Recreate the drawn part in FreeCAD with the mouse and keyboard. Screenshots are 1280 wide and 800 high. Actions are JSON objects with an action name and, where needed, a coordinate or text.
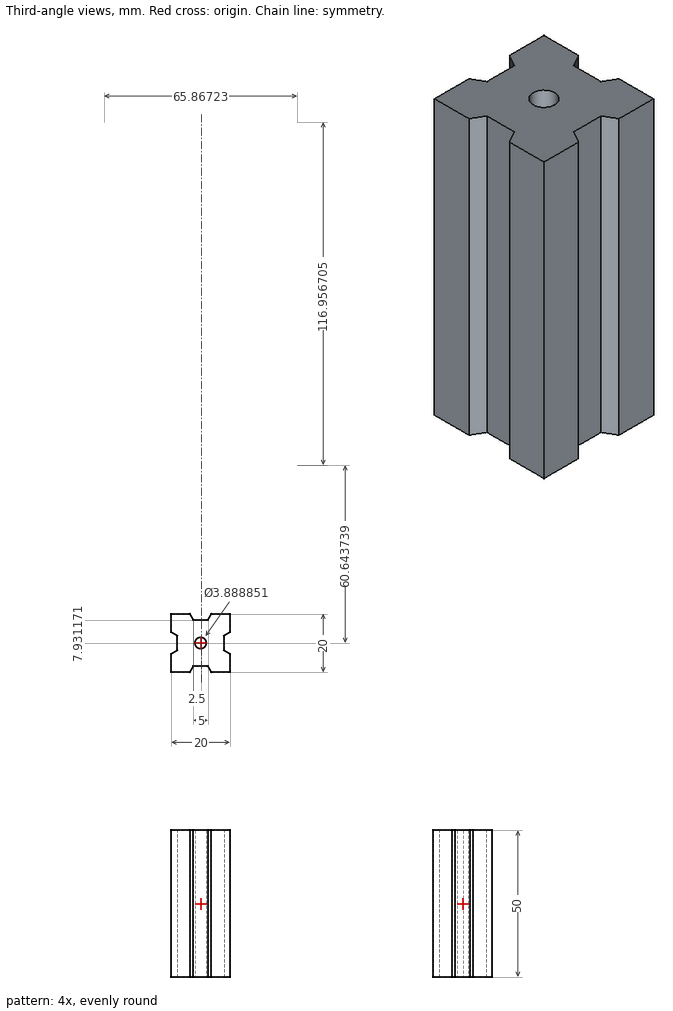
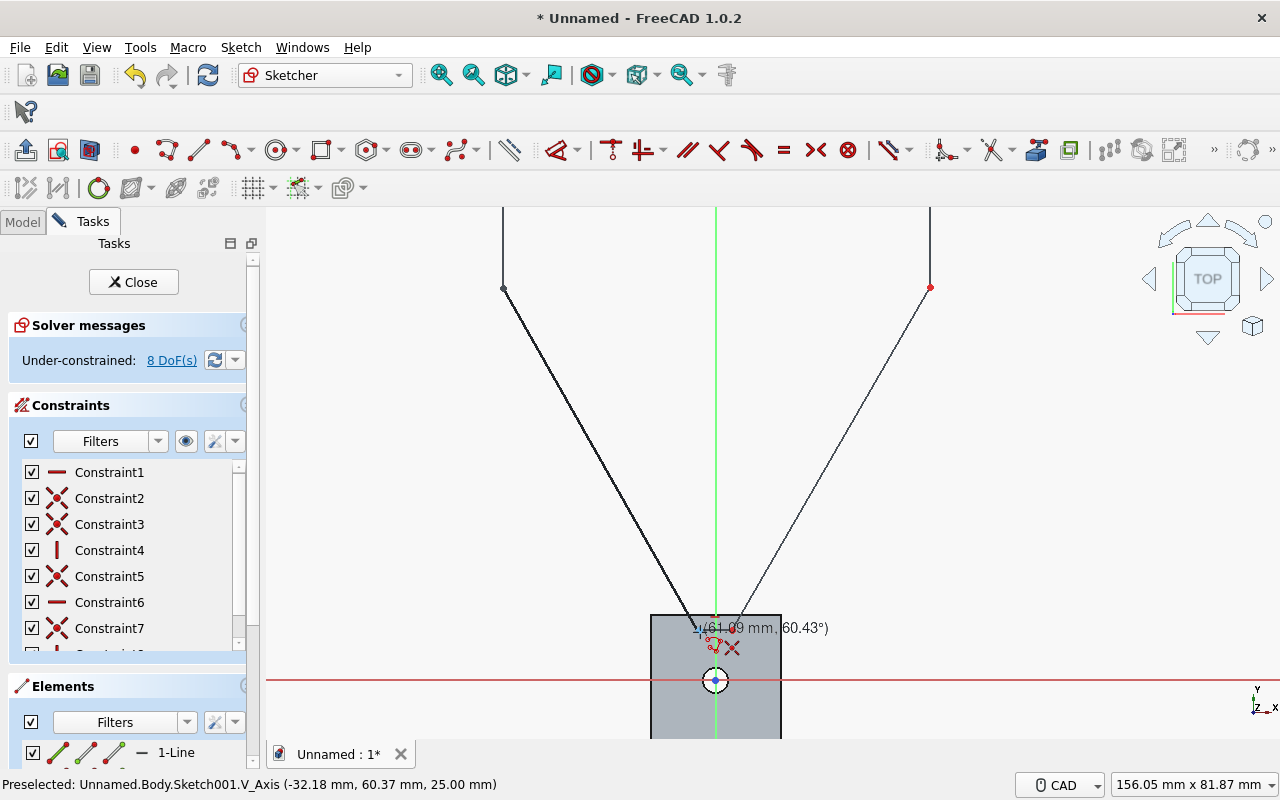
{"action": "left_click", "coordinate": [699, 630]}
{"action": "key", "text": "Escape"}
{"action": "key", "text": "Escape"}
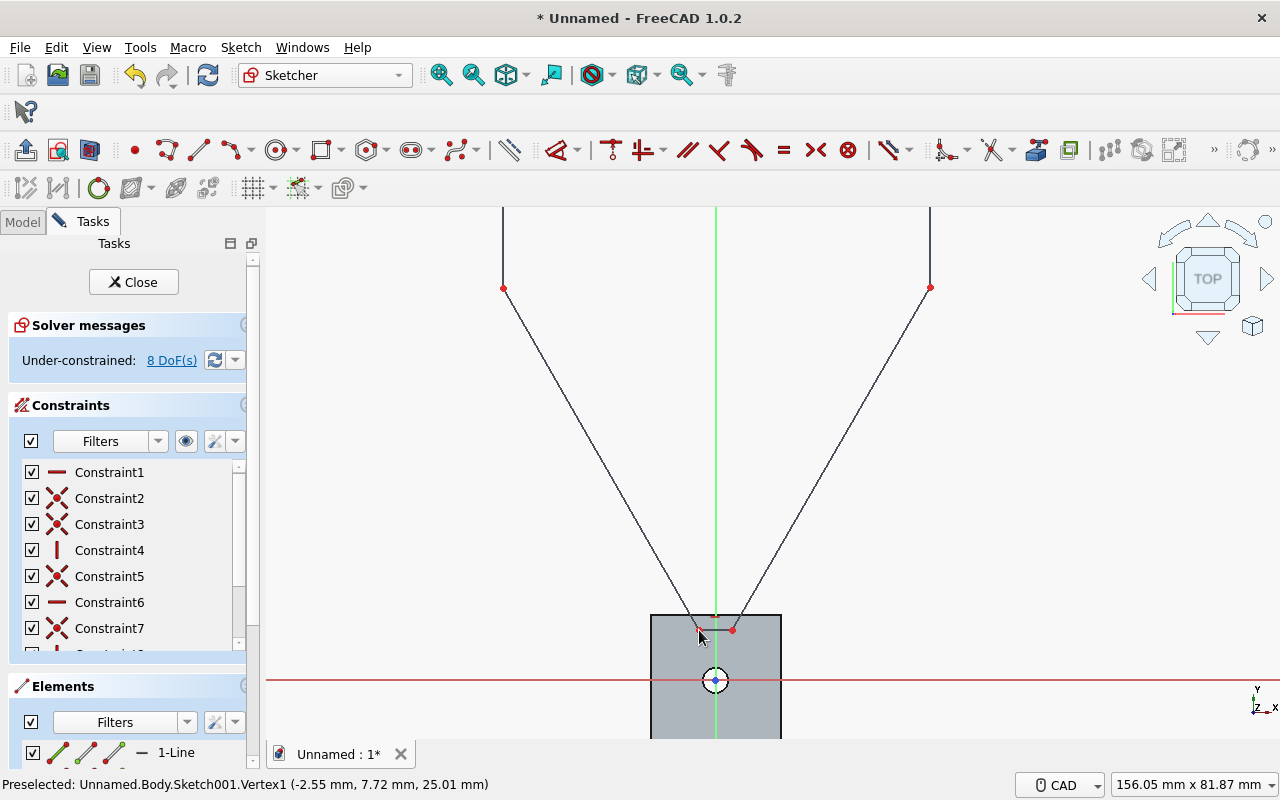
{"action": "left_click", "coordinate": [930, 287]}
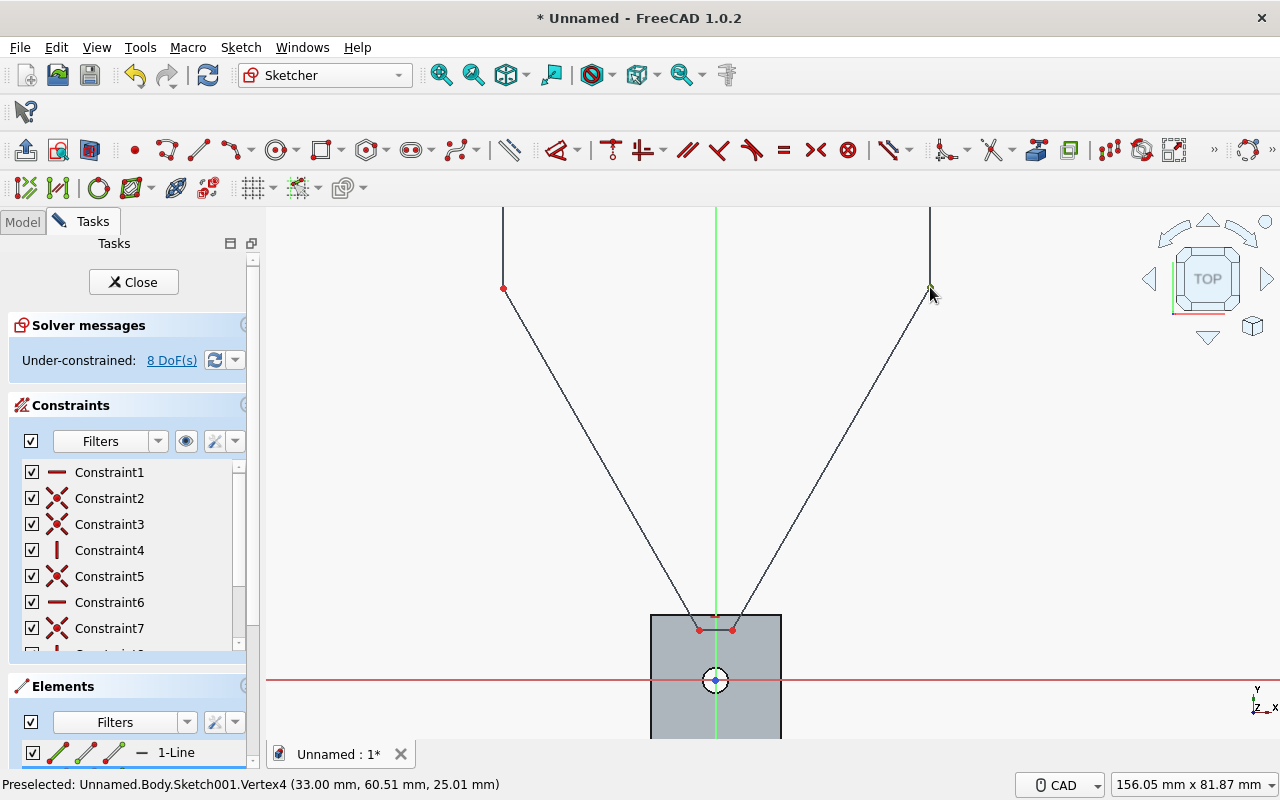
{"action": "left_click", "coordinate": [503, 288]}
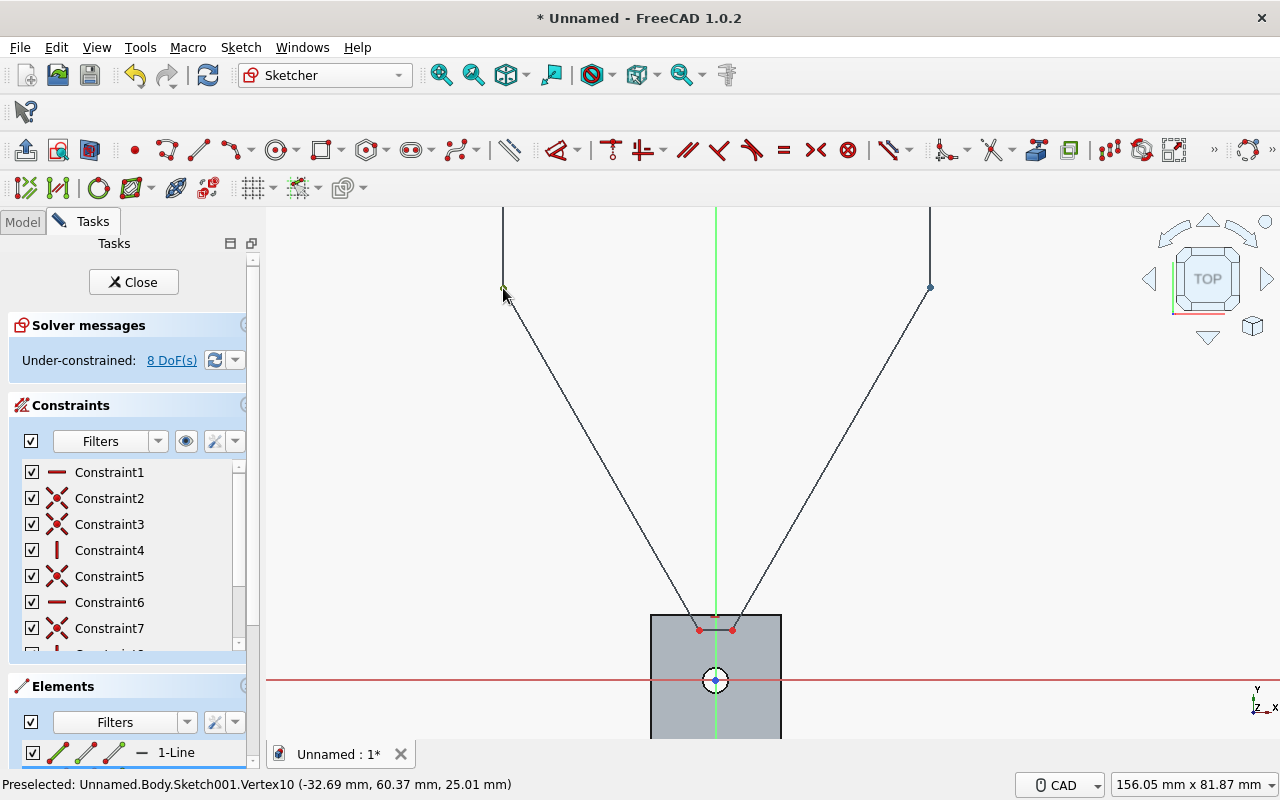
{"action": "left_click", "coordinate": [716, 575]}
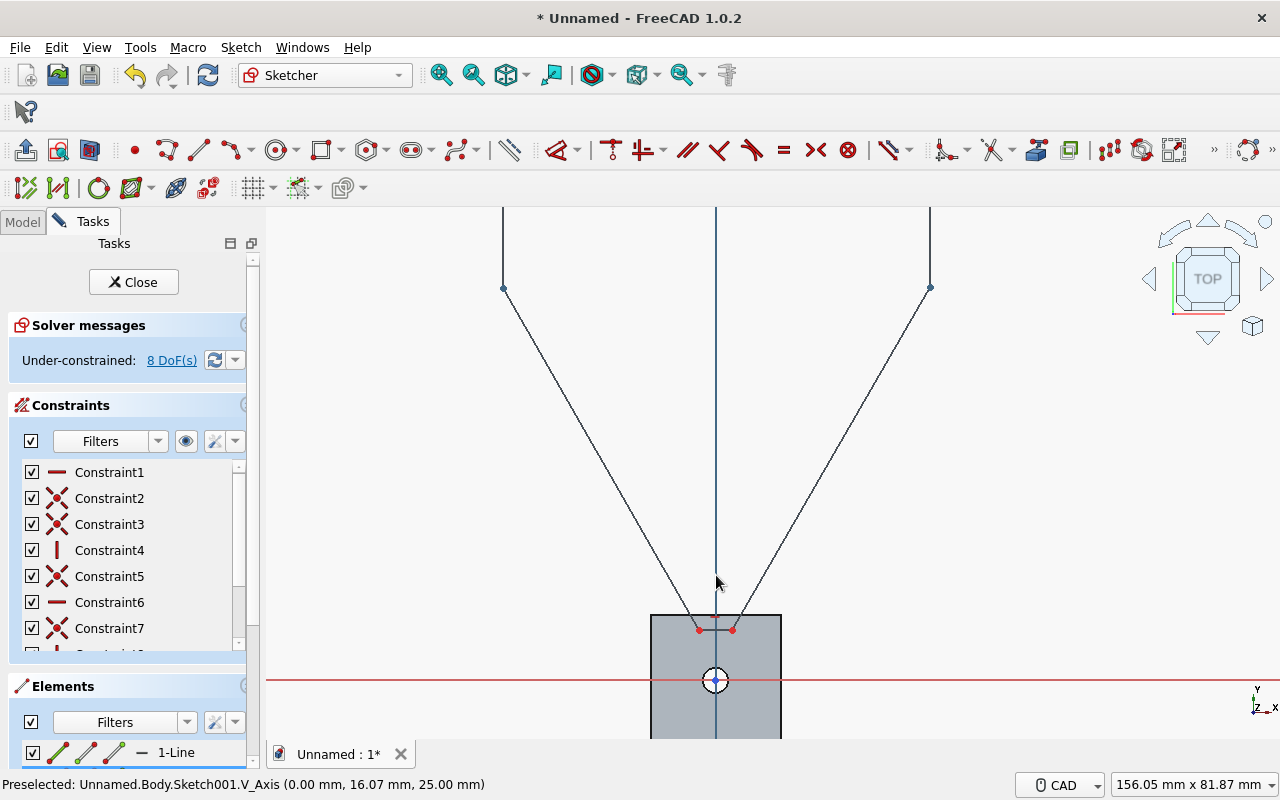
{"action": "key", "text": "s"}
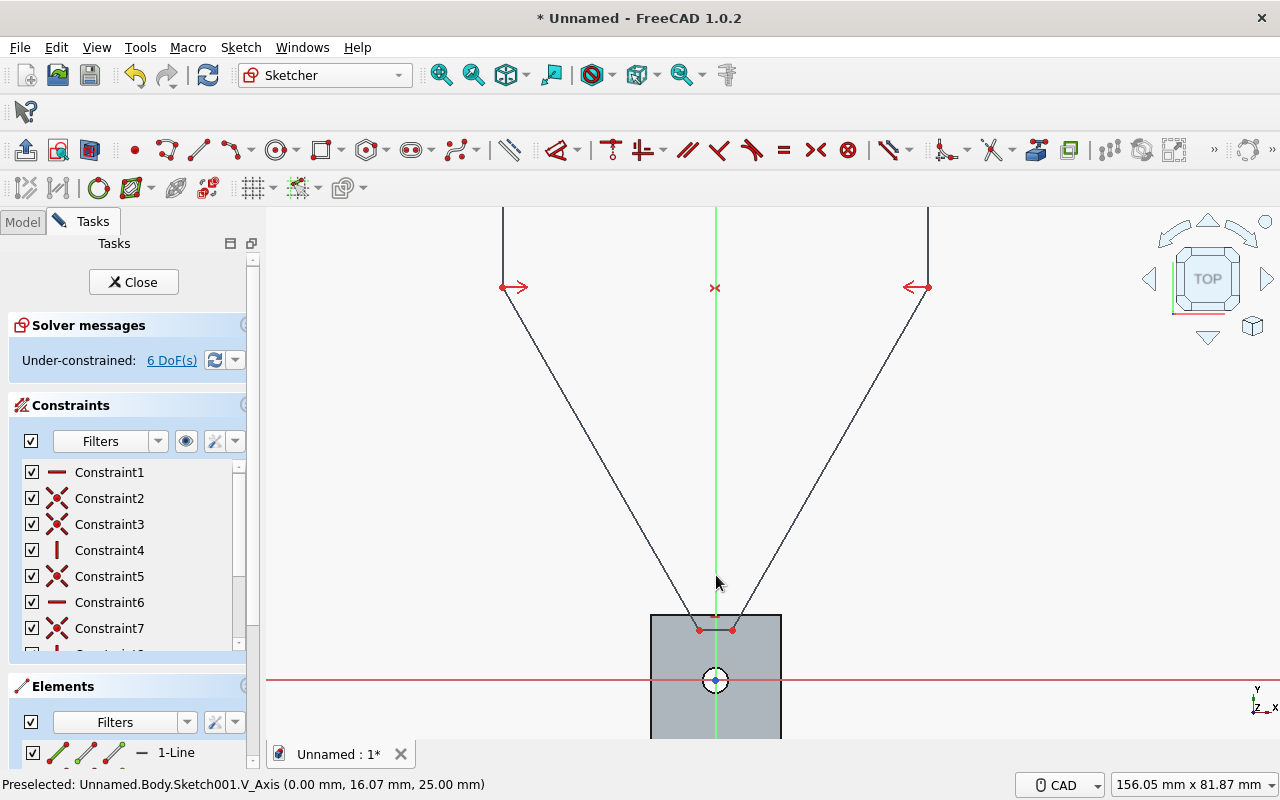
{"action": "left_click", "coordinate": [556, 150]}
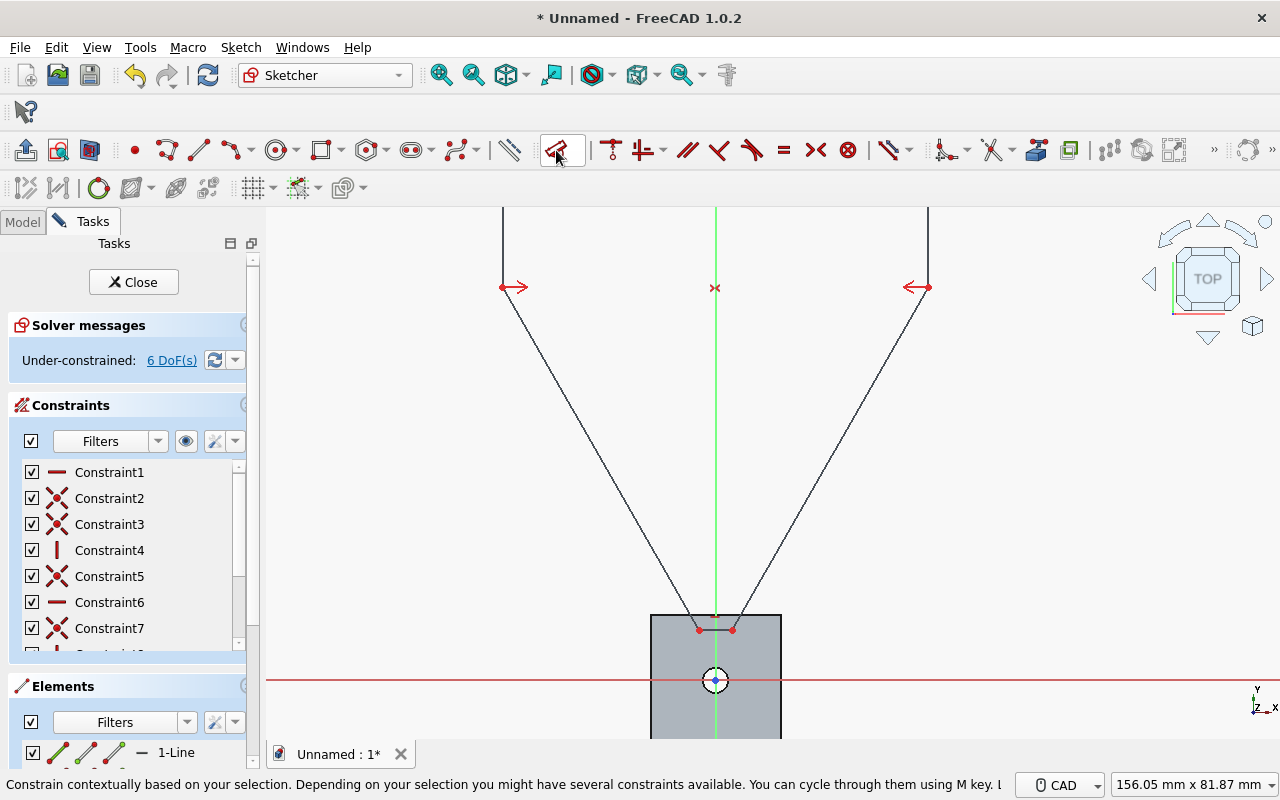
{"action": "scroll", "coordinate": [712, 630], "scroll_direction": "up", "scroll_amount": 2}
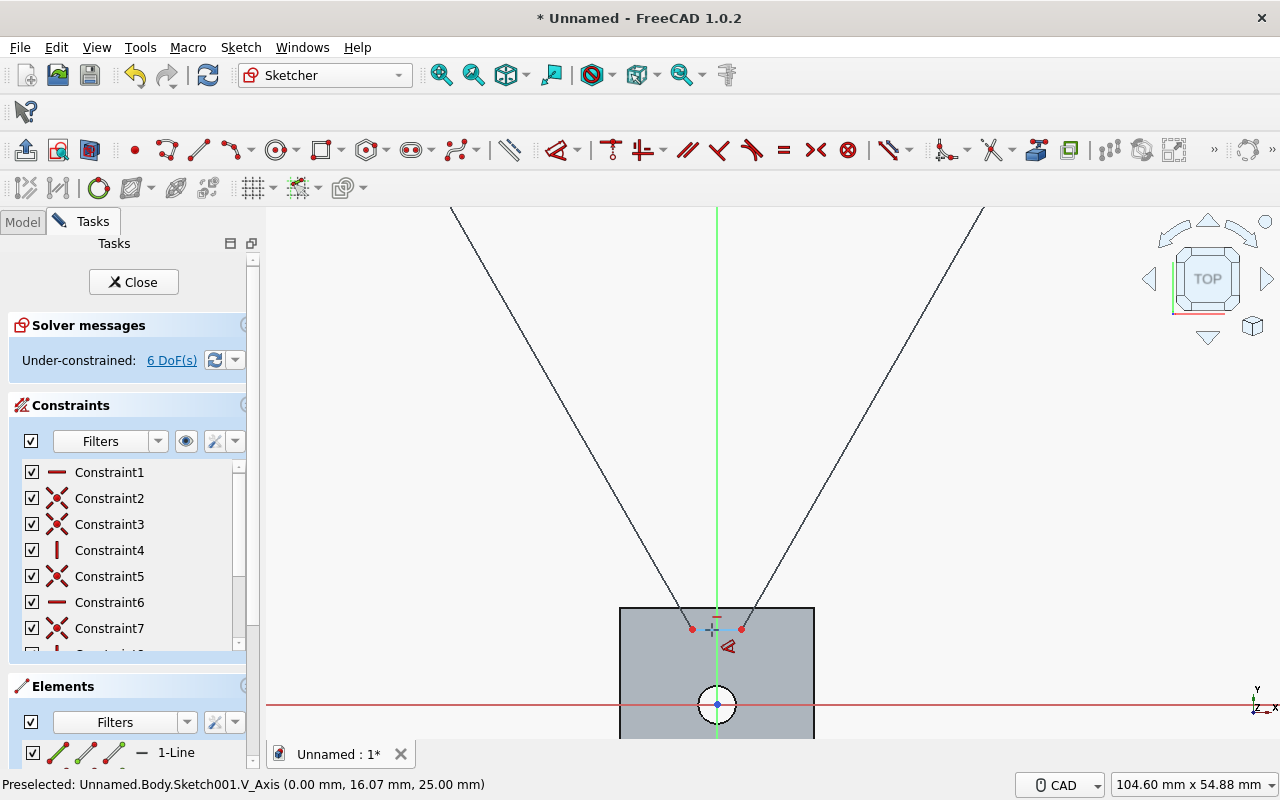
{"action": "left_click", "coordinate": [712, 630]}
{"action": "left_click", "coordinate": [700, 664]}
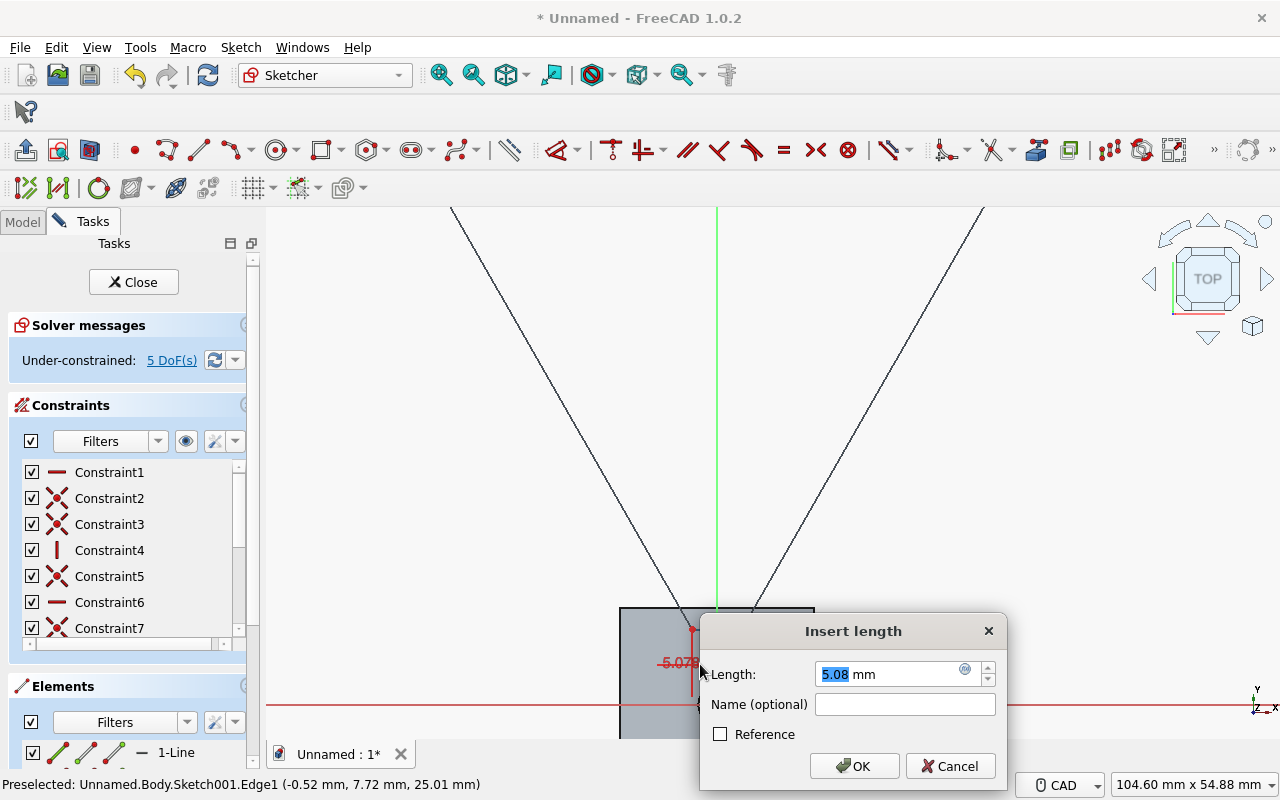
{"action": "type", "text": "5"}
{"action": "key", "text": "Return"}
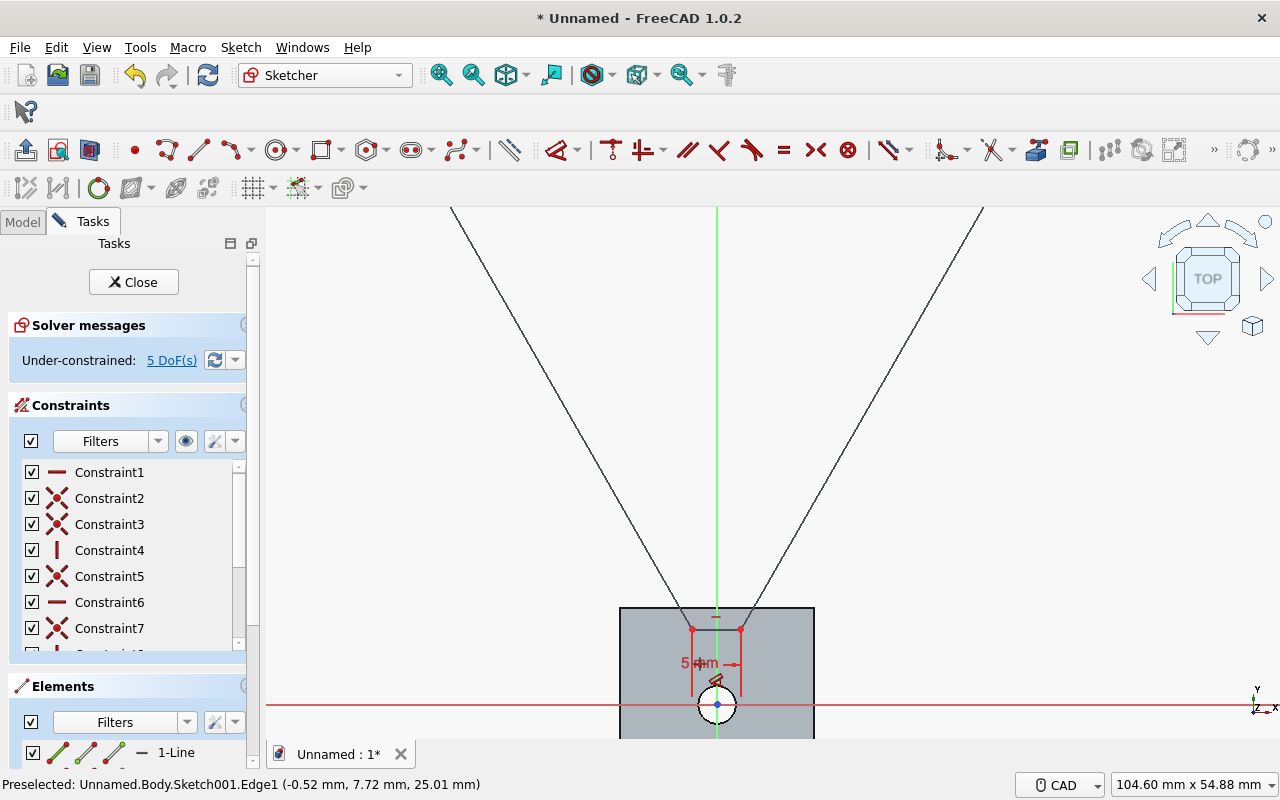
{"action": "scroll", "coordinate": [692, 630], "scroll_direction": "up", "scroll_amount": 3}